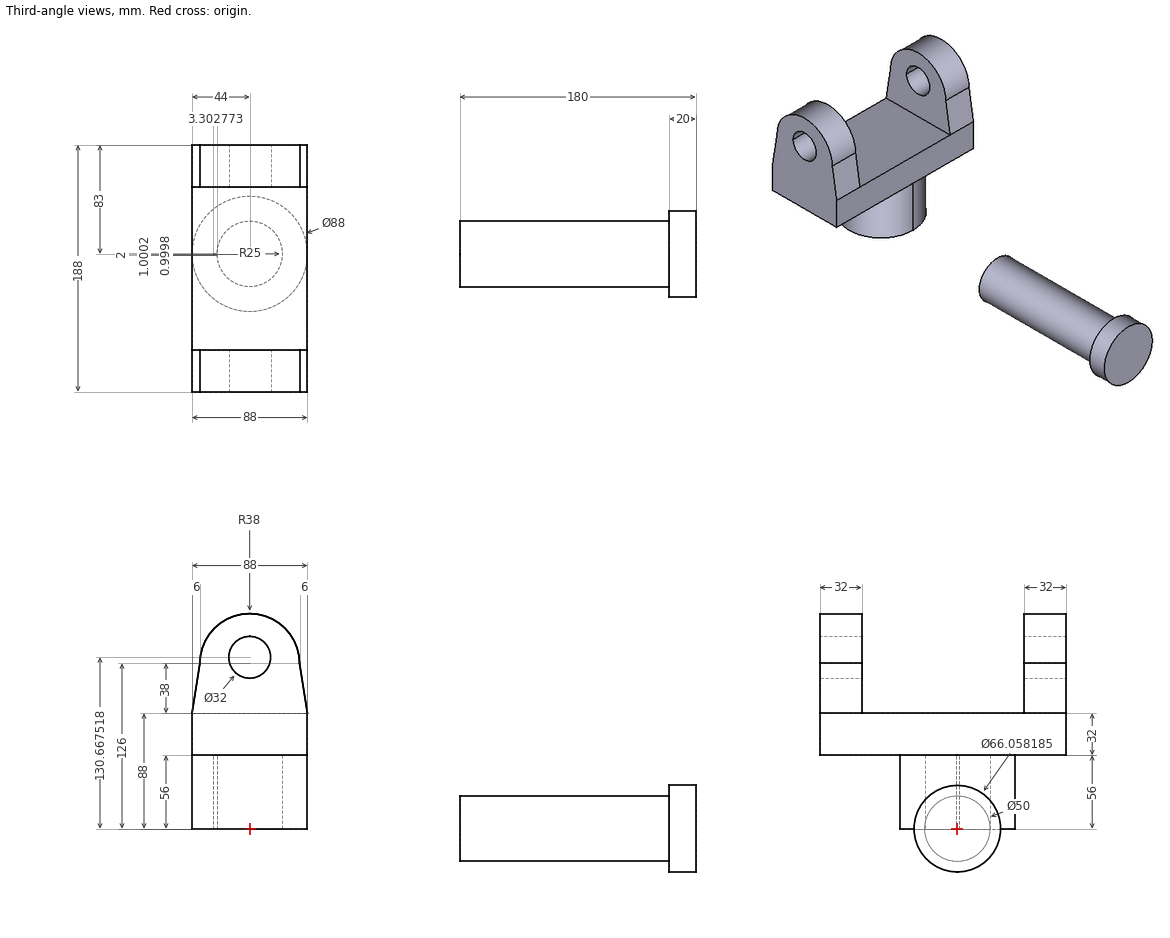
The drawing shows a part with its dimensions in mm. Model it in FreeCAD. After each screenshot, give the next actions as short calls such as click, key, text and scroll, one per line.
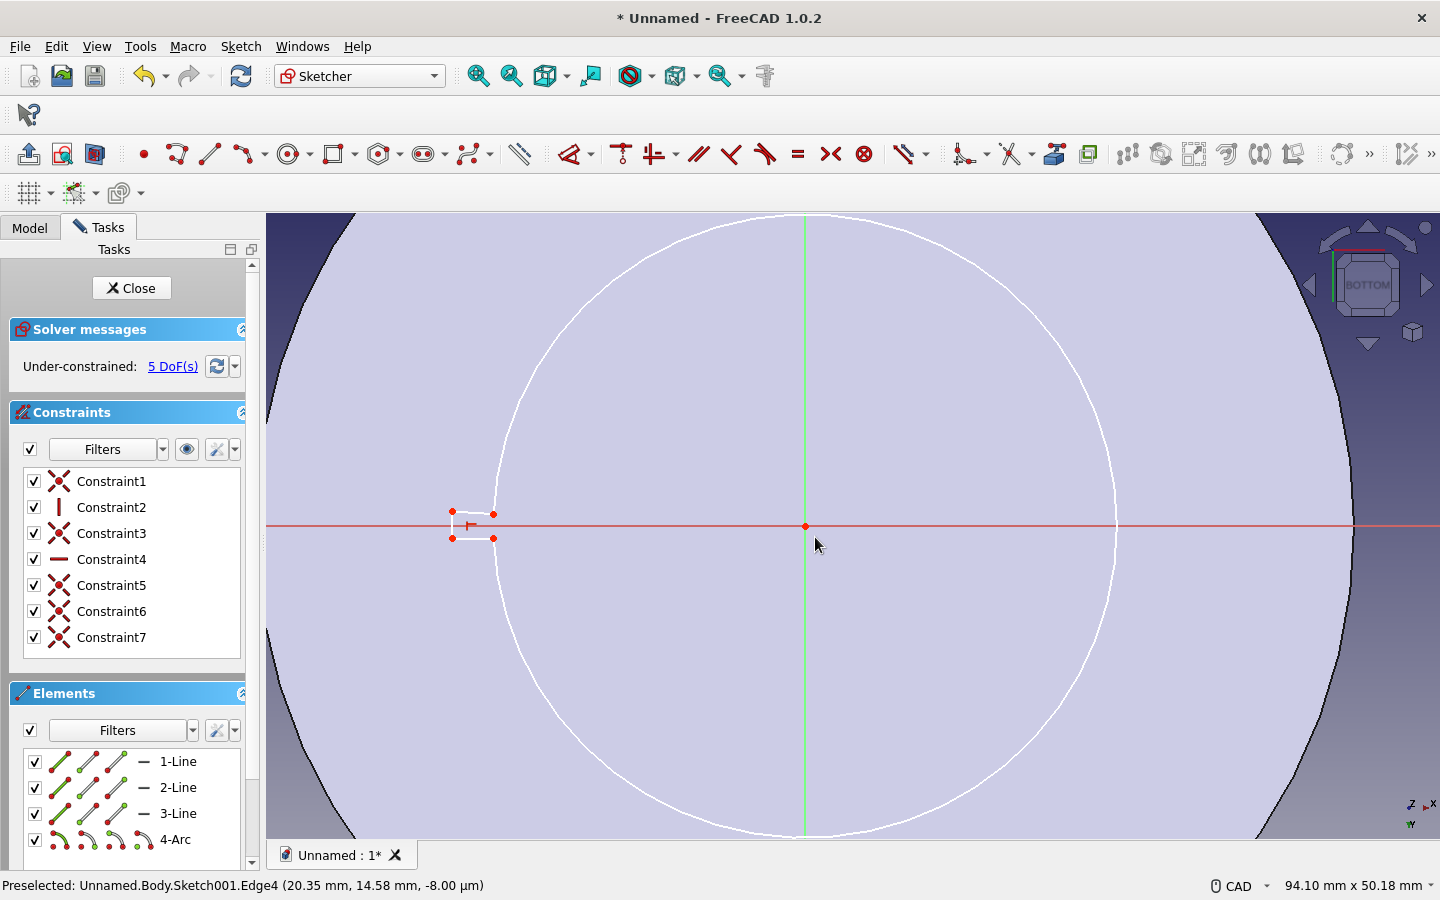
key(d)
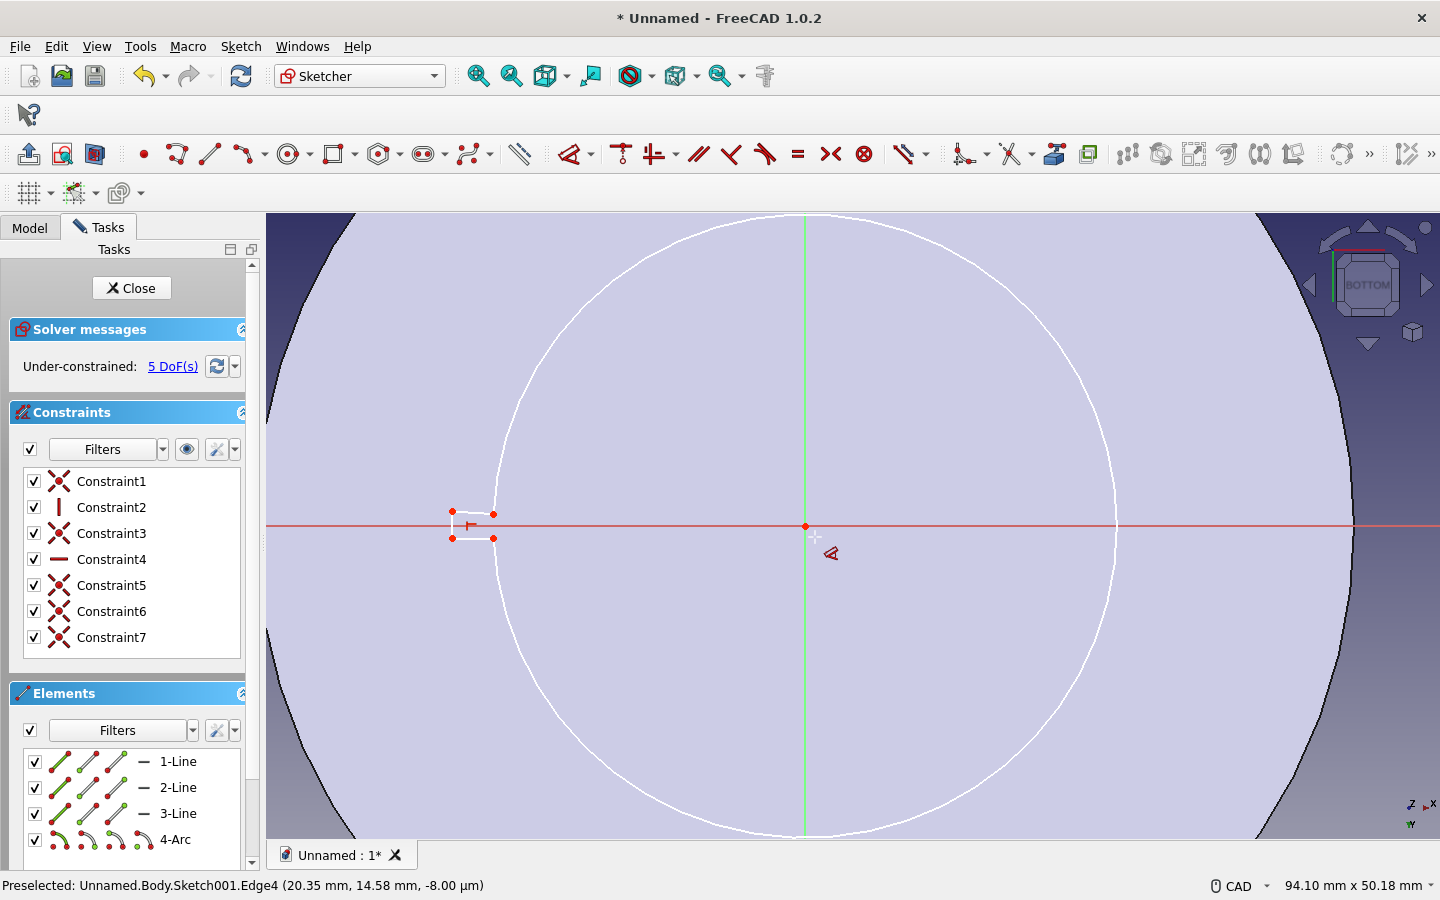
click(1117, 526)
click(1107, 691)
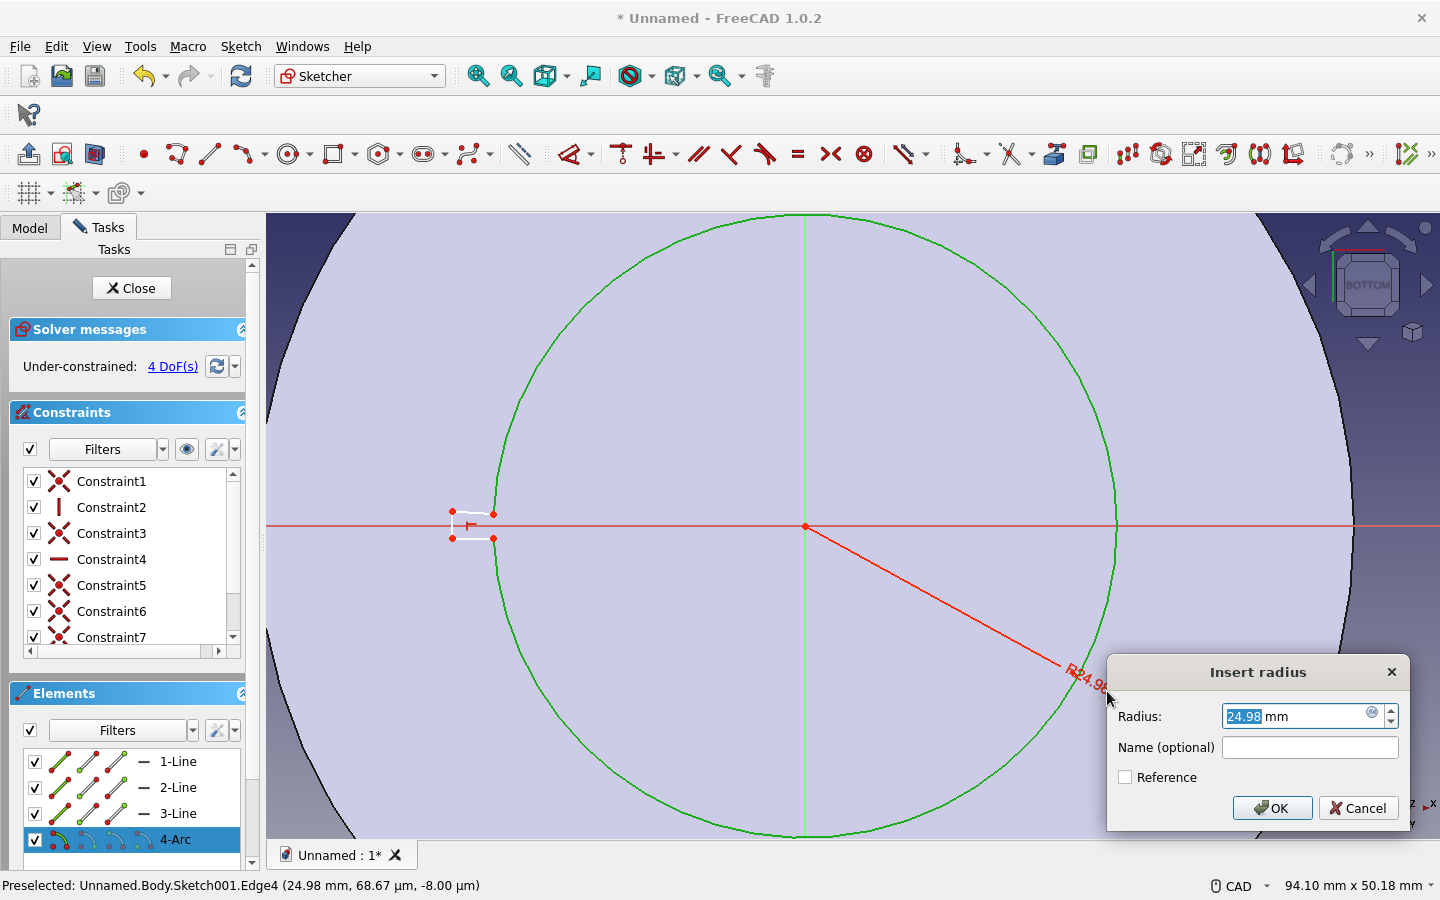
text(25)
key(Return)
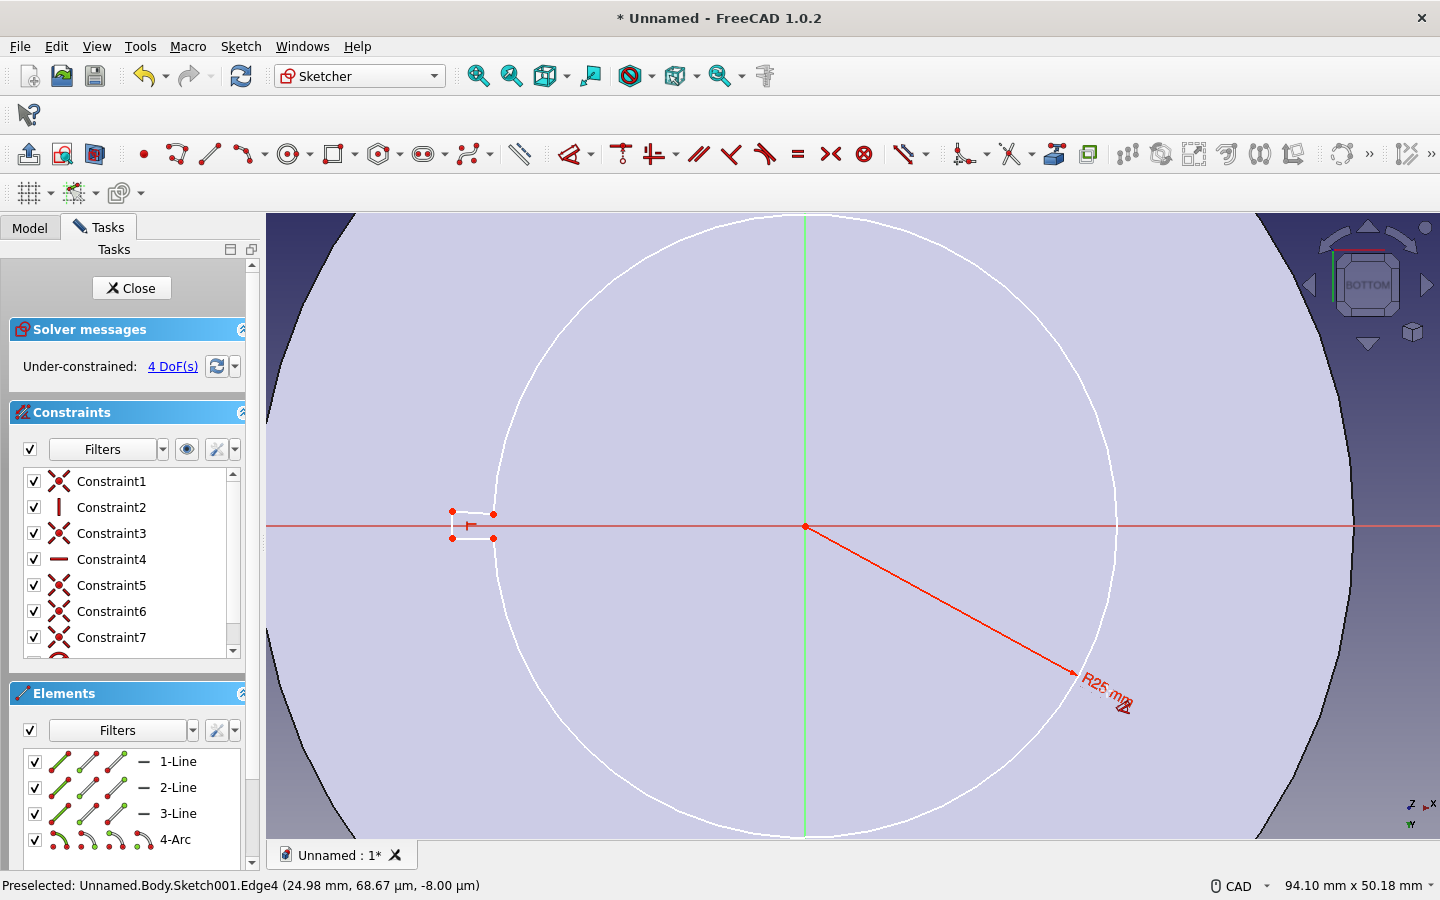
scroll(452, 522, up, 3)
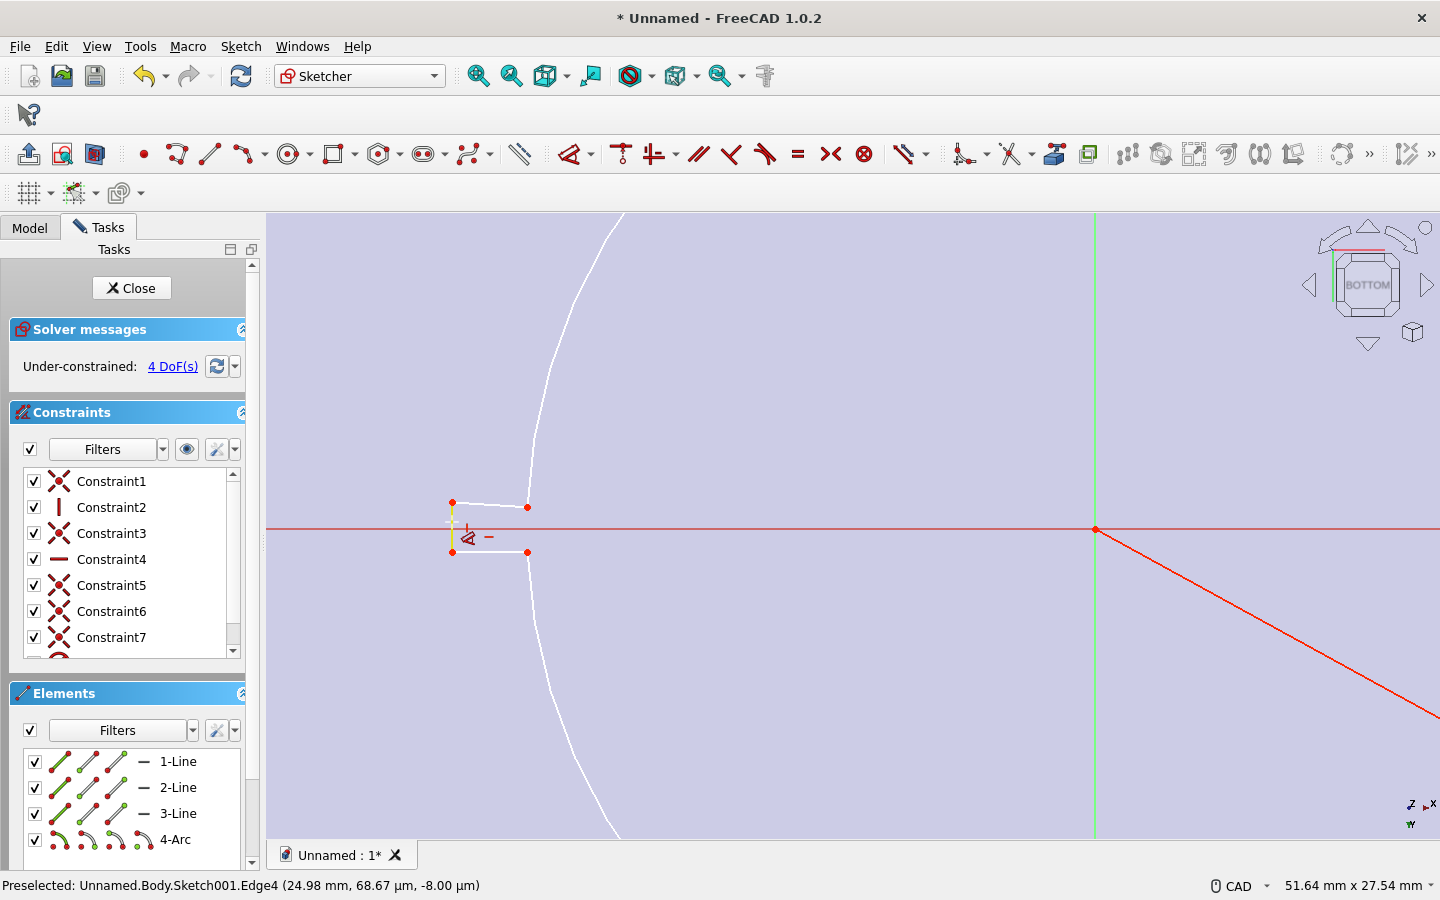
click(452, 522)
click(418, 516)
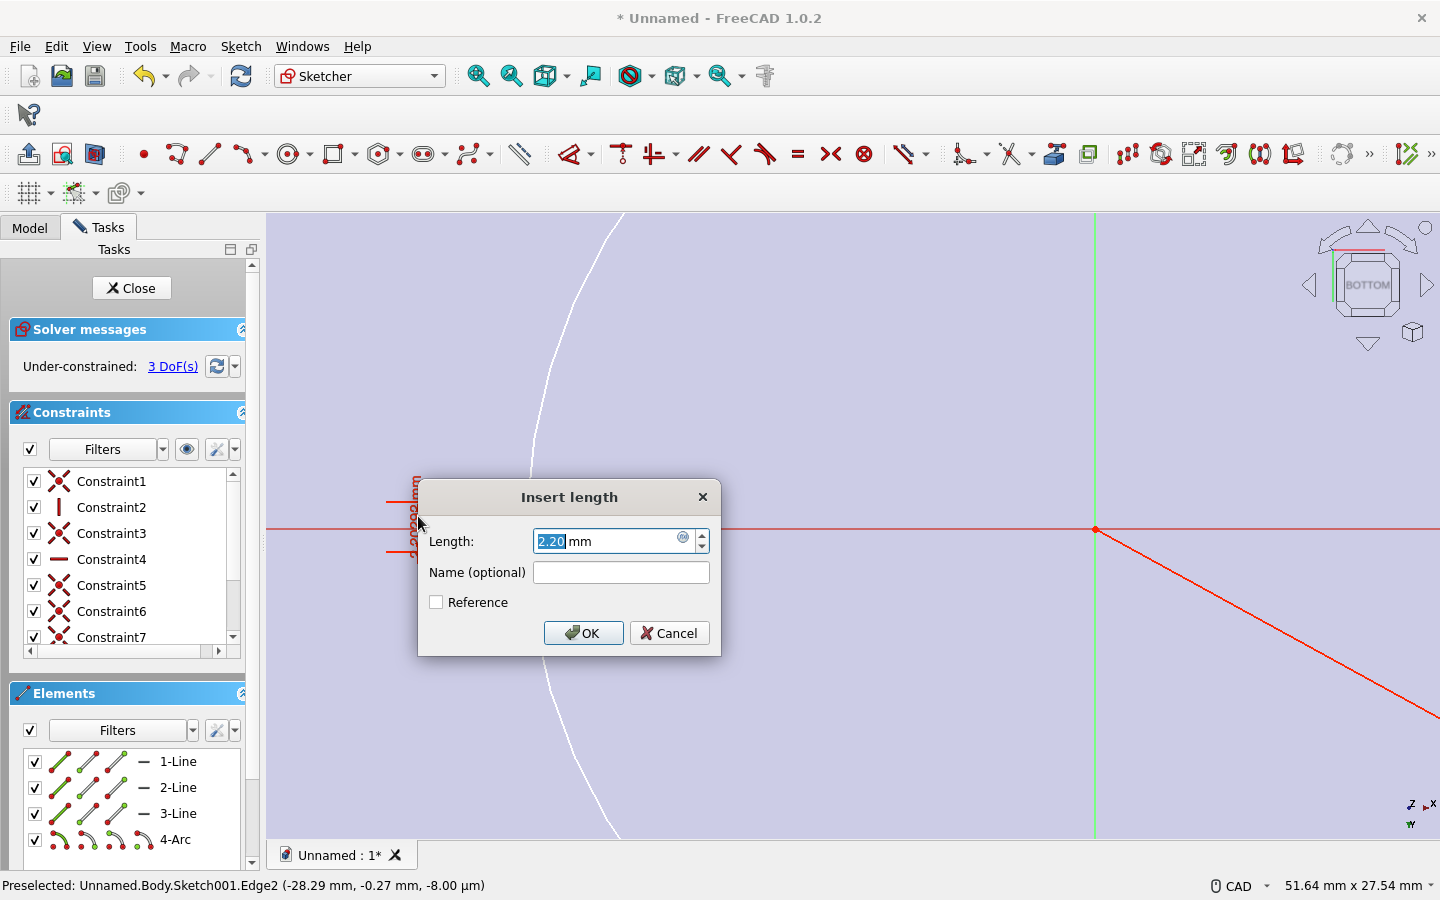
text(2)
key(Return)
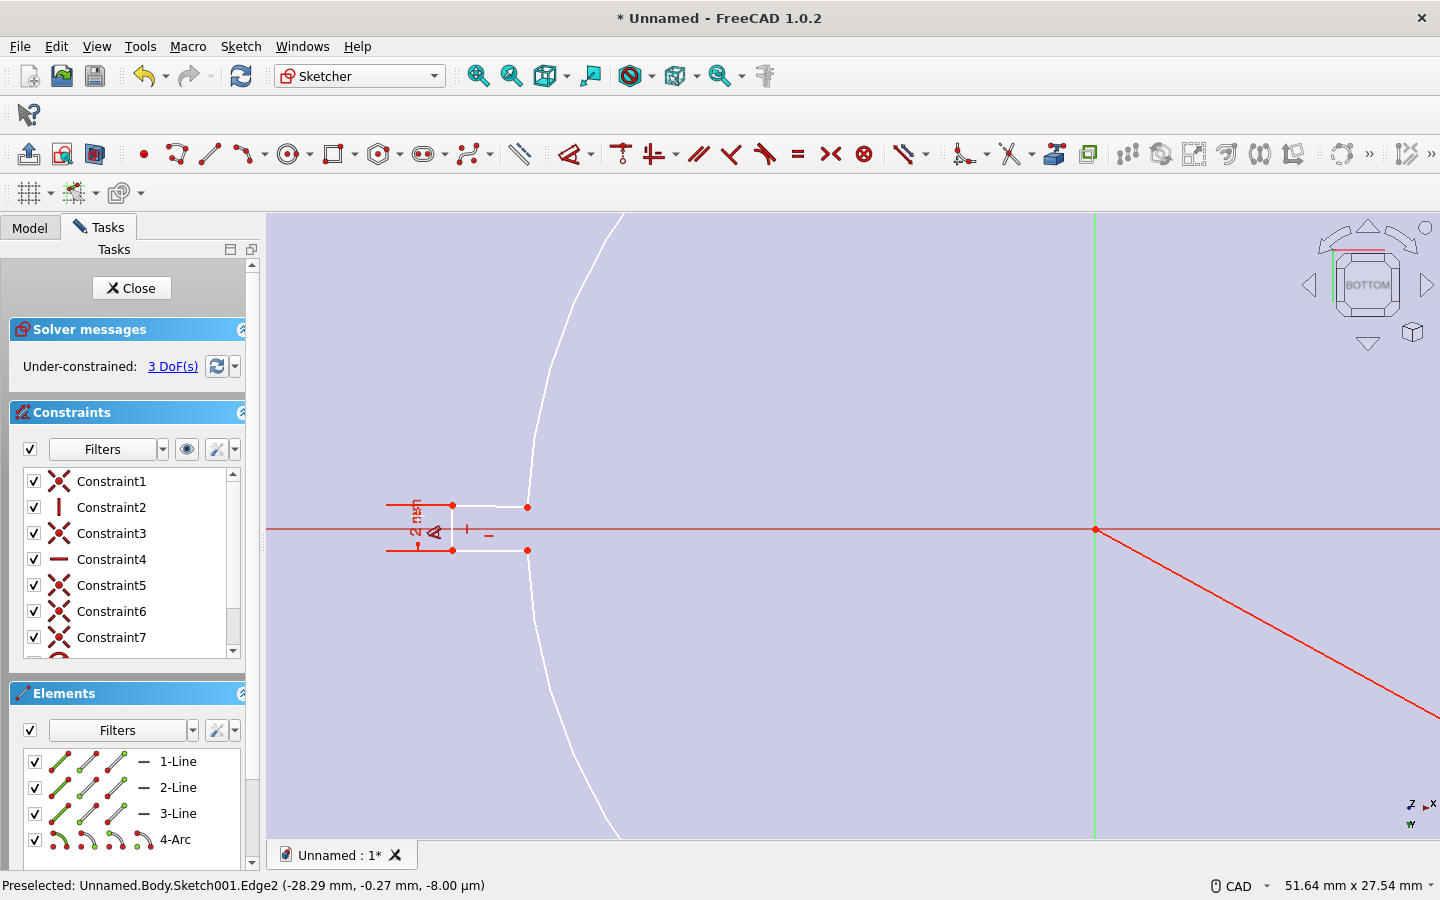
scroll(527, 507, up, 3)